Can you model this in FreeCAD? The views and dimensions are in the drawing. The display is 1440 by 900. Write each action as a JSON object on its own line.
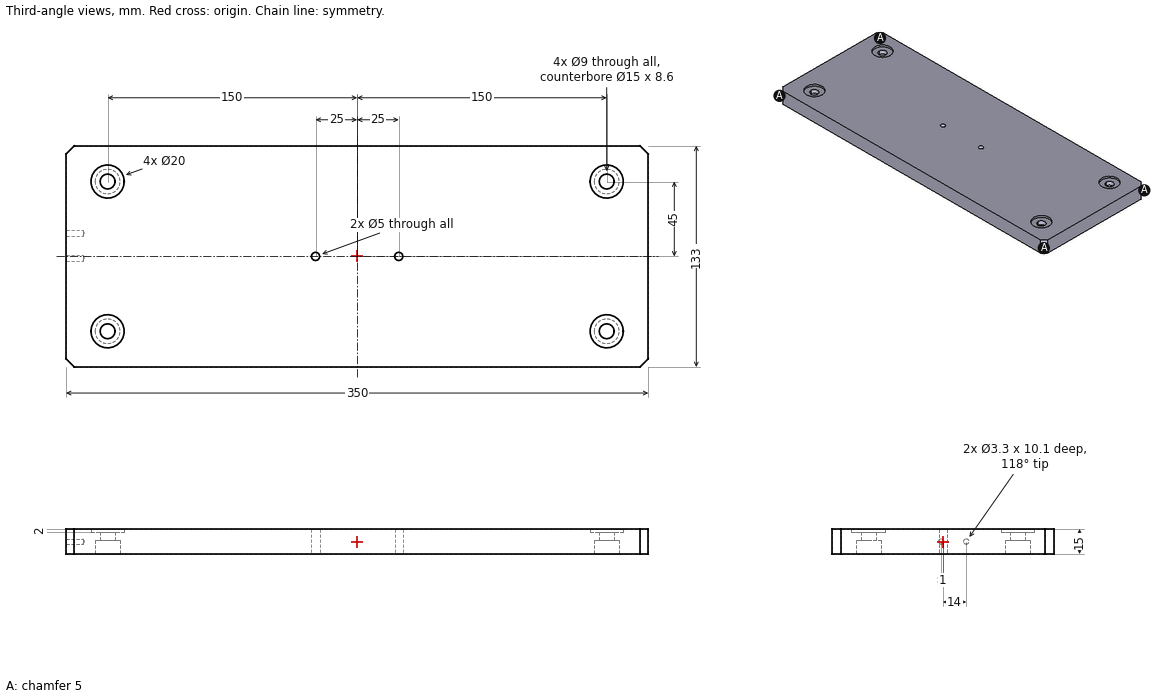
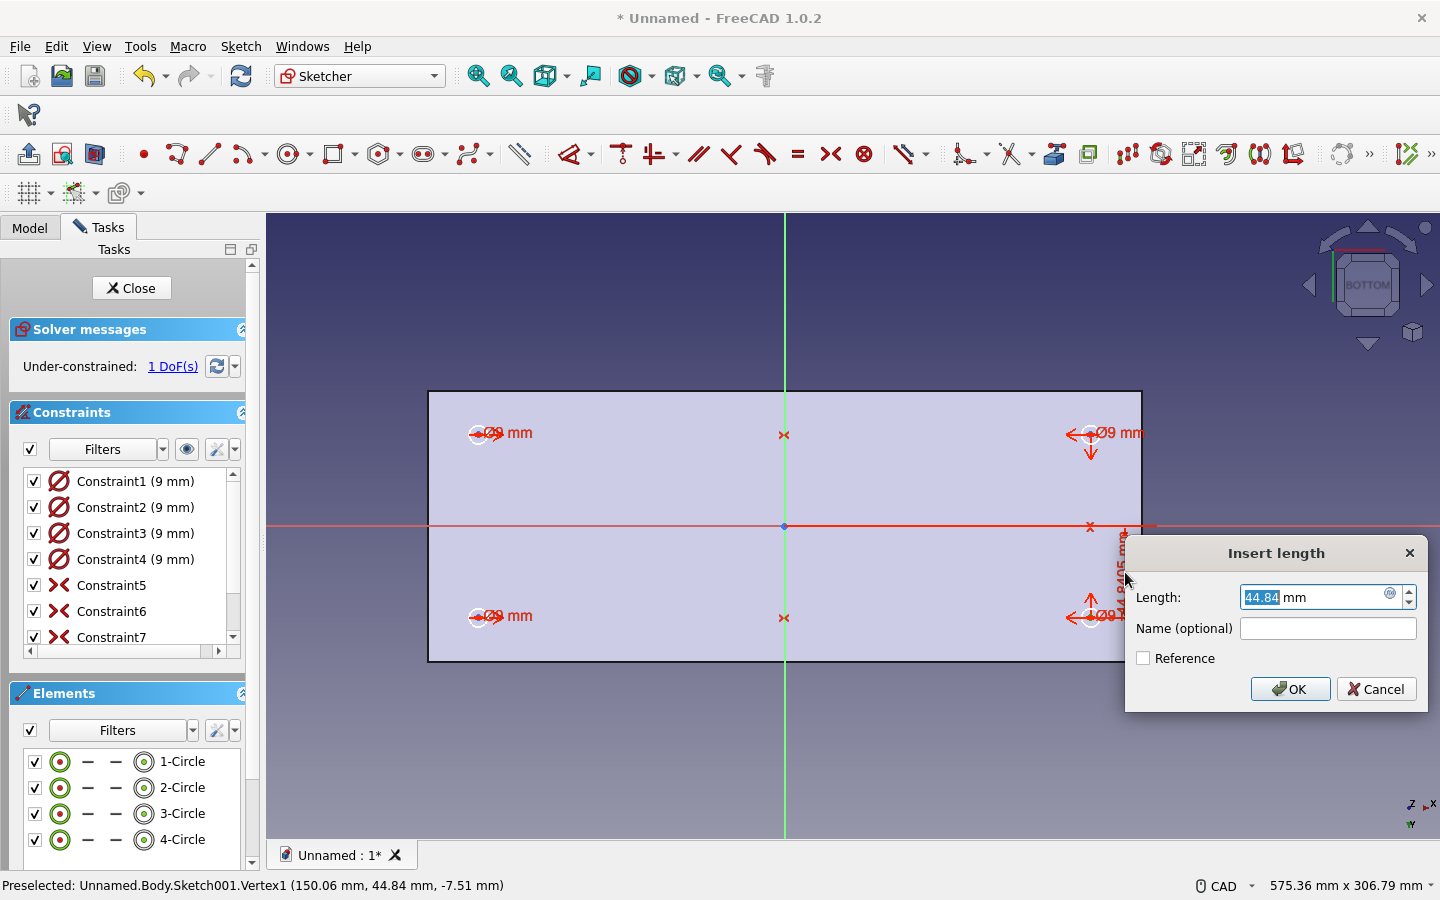
{"action": "type", "text": "45"}
{"action": "key", "text": "Return"}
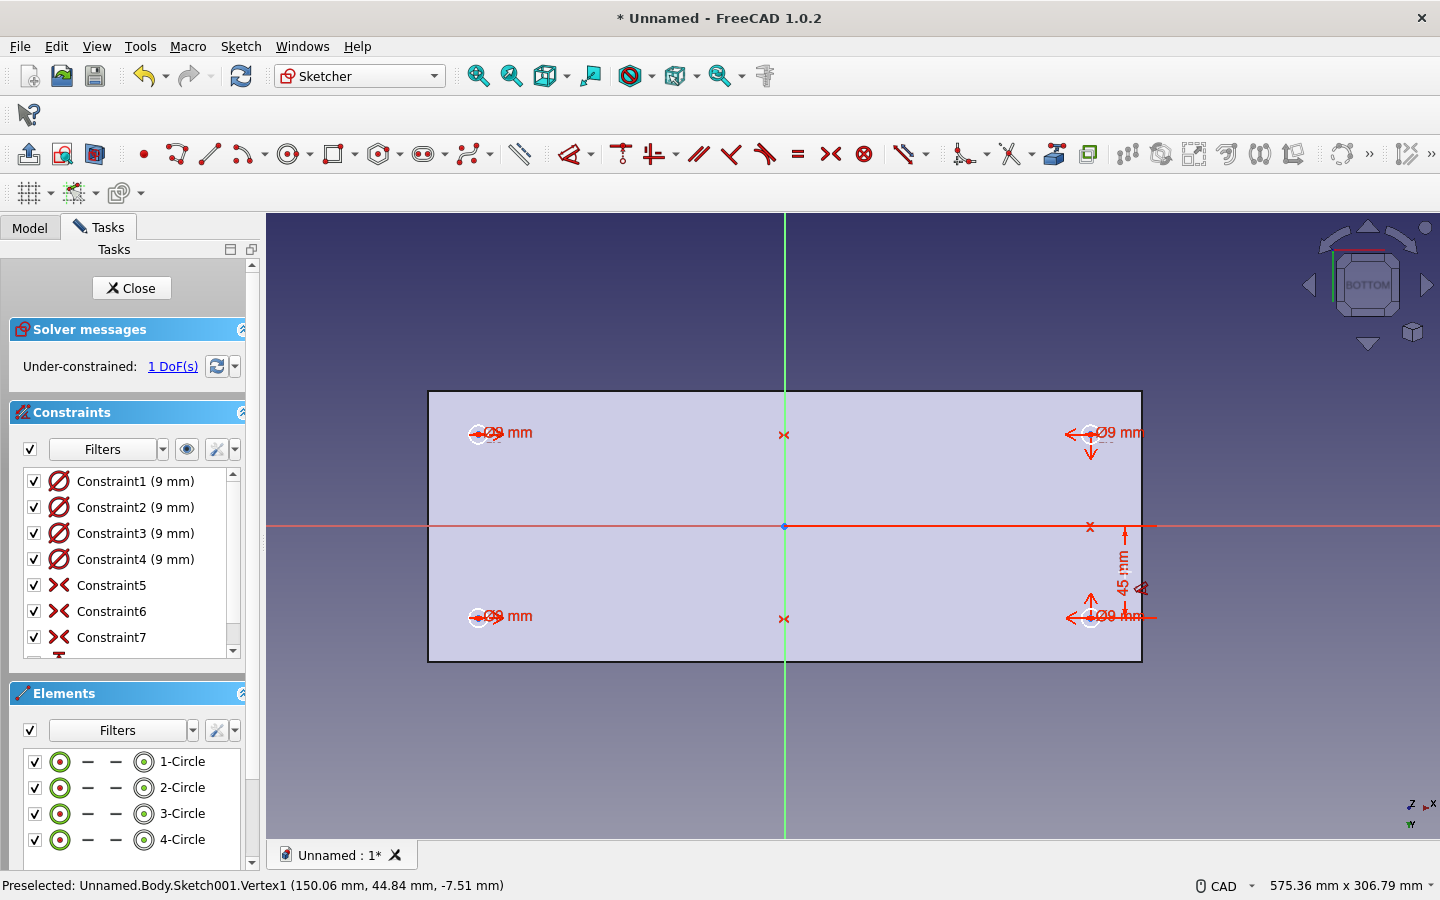
{"action": "left_click", "coordinate": [1091, 618]}
{"action": "left_click", "coordinate": [938, 652]}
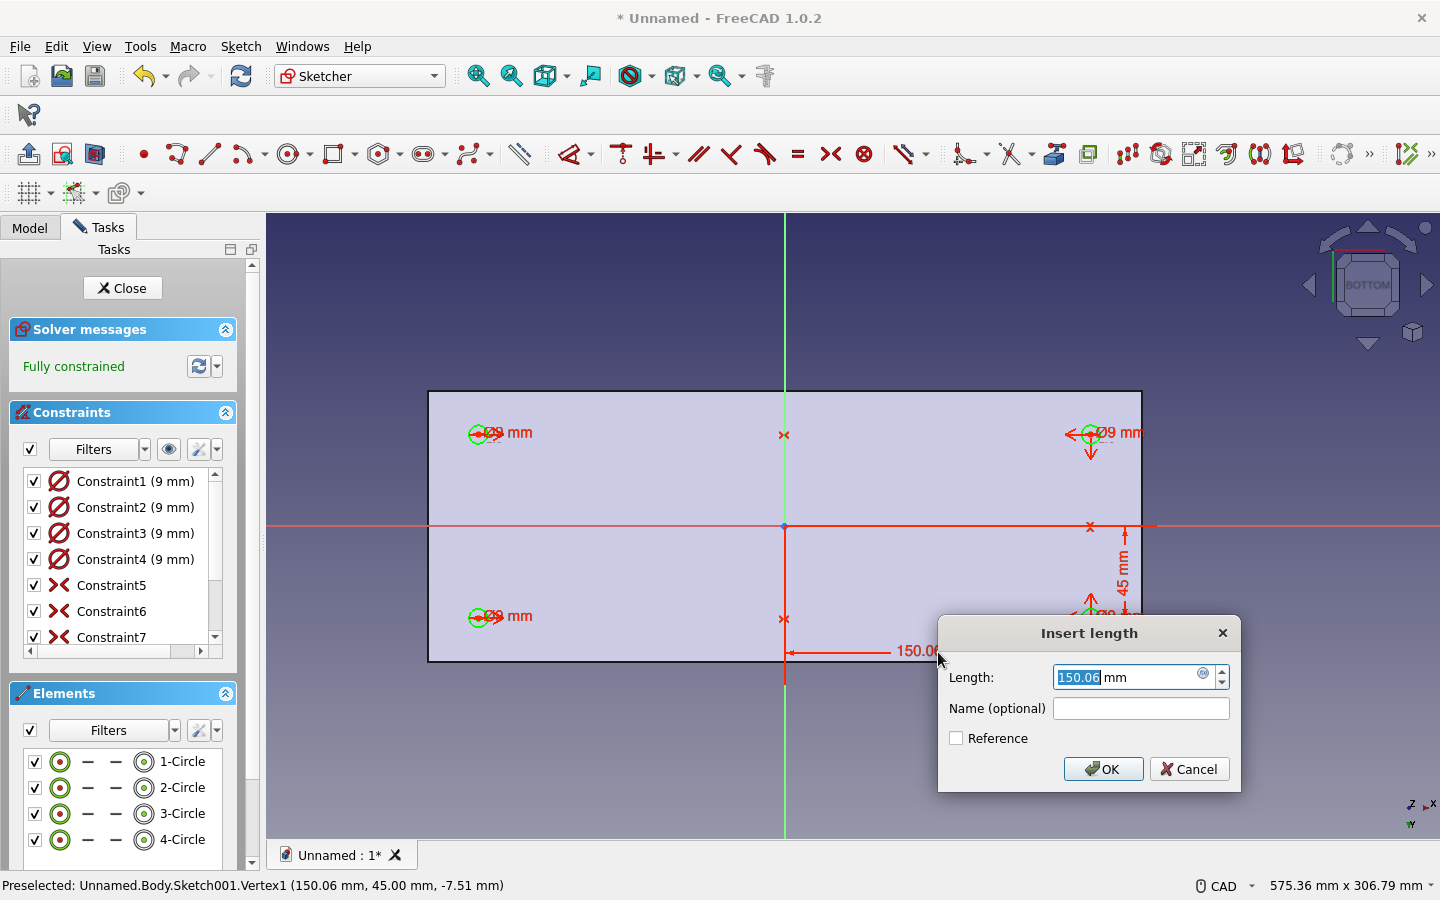
{"action": "type", "text": "150"}
{"action": "key", "text": "Return"}
{"action": "key", "text": "Escape"}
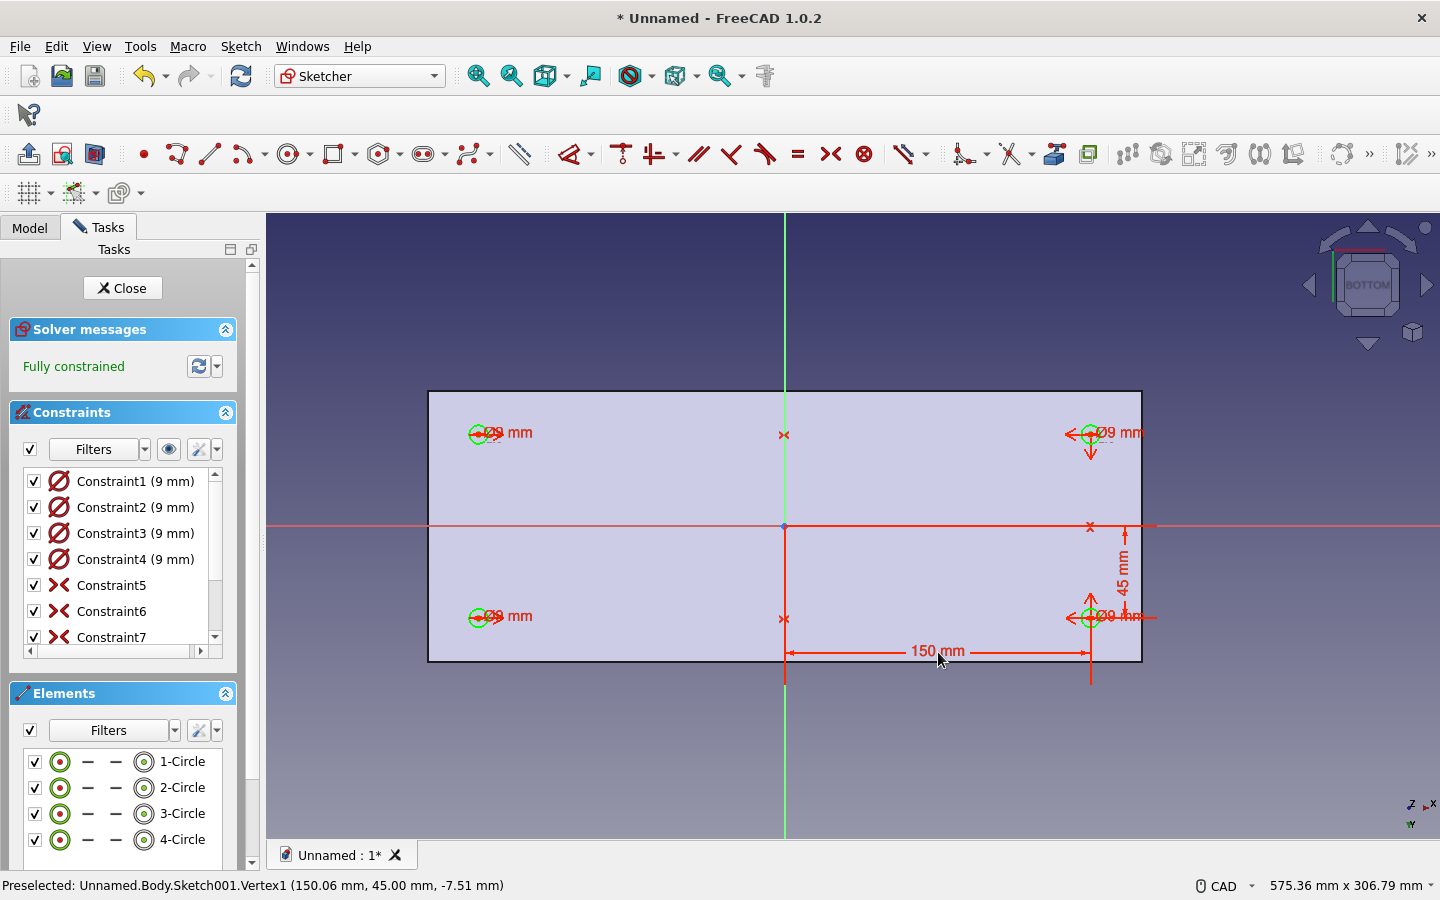
{"action": "left_click", "coordinate": [123, 288]}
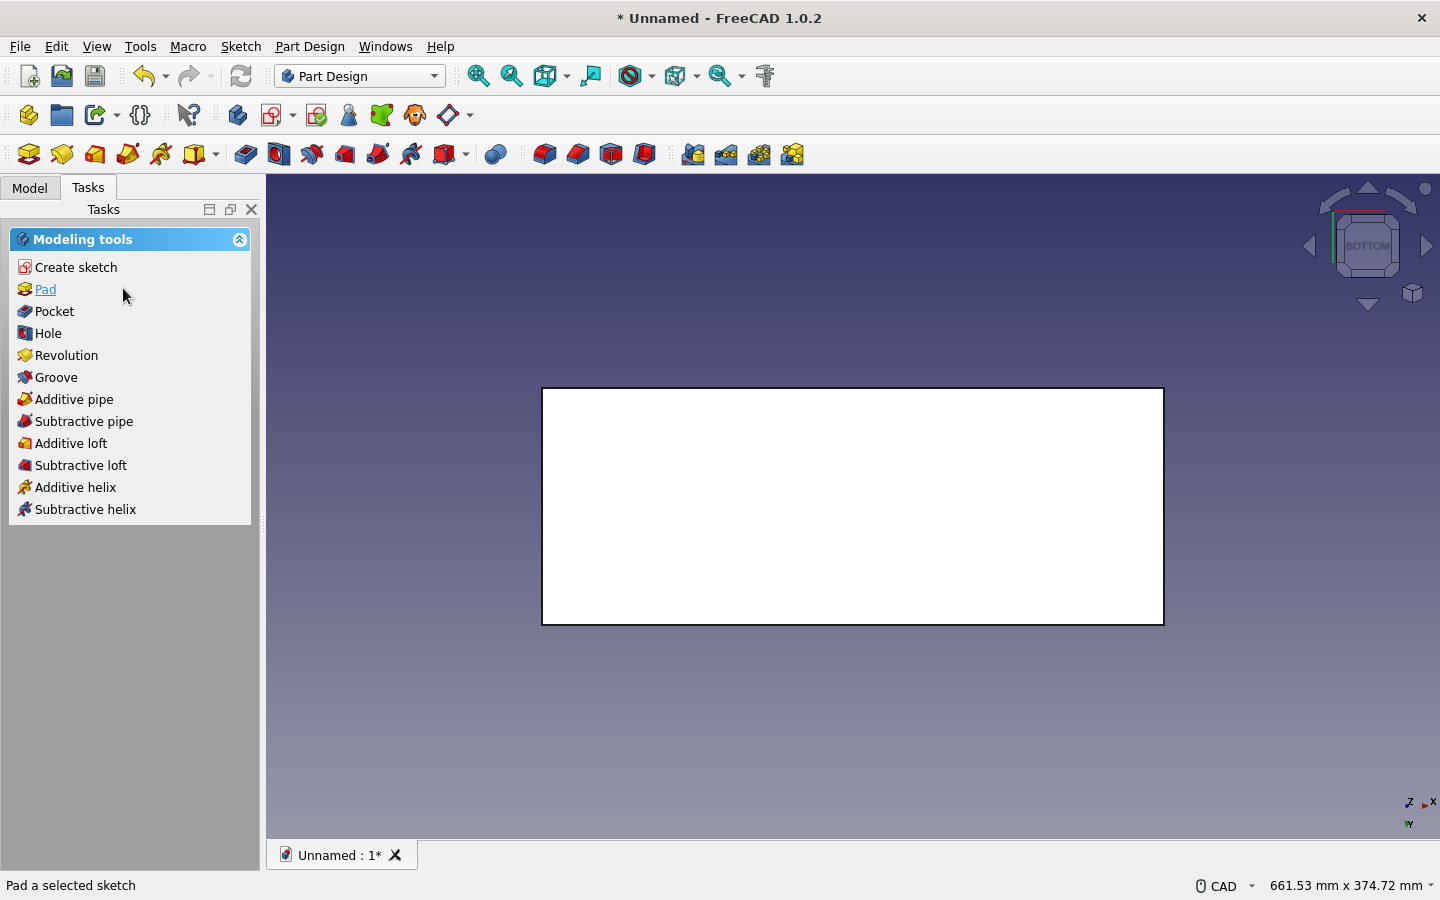
{"action": "left_click", "coordinate": [279, 154]}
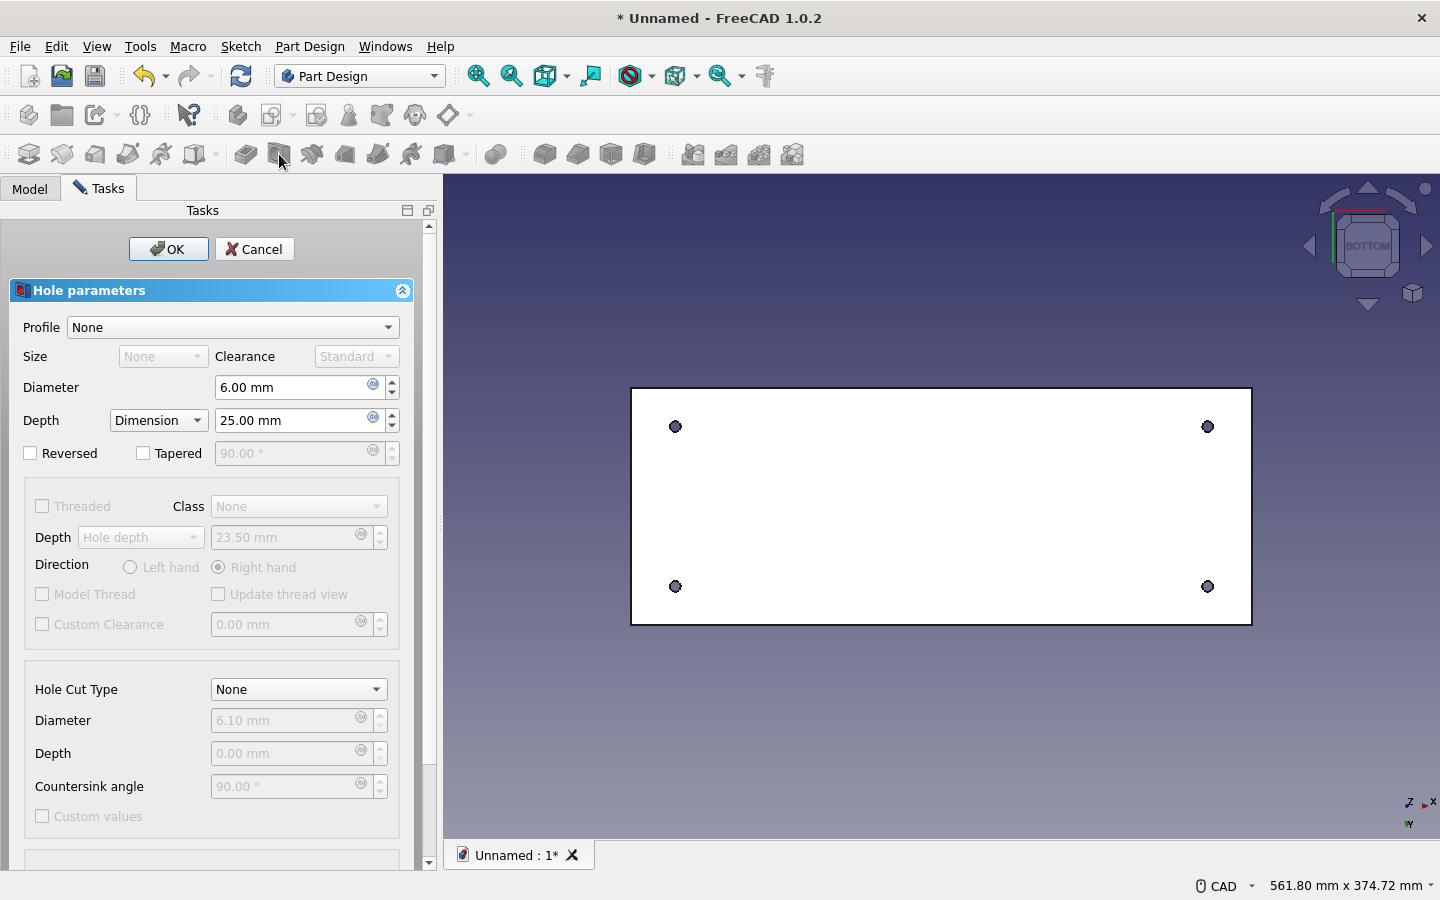
{"action": "triple_click", "coordinate": [300, 388]}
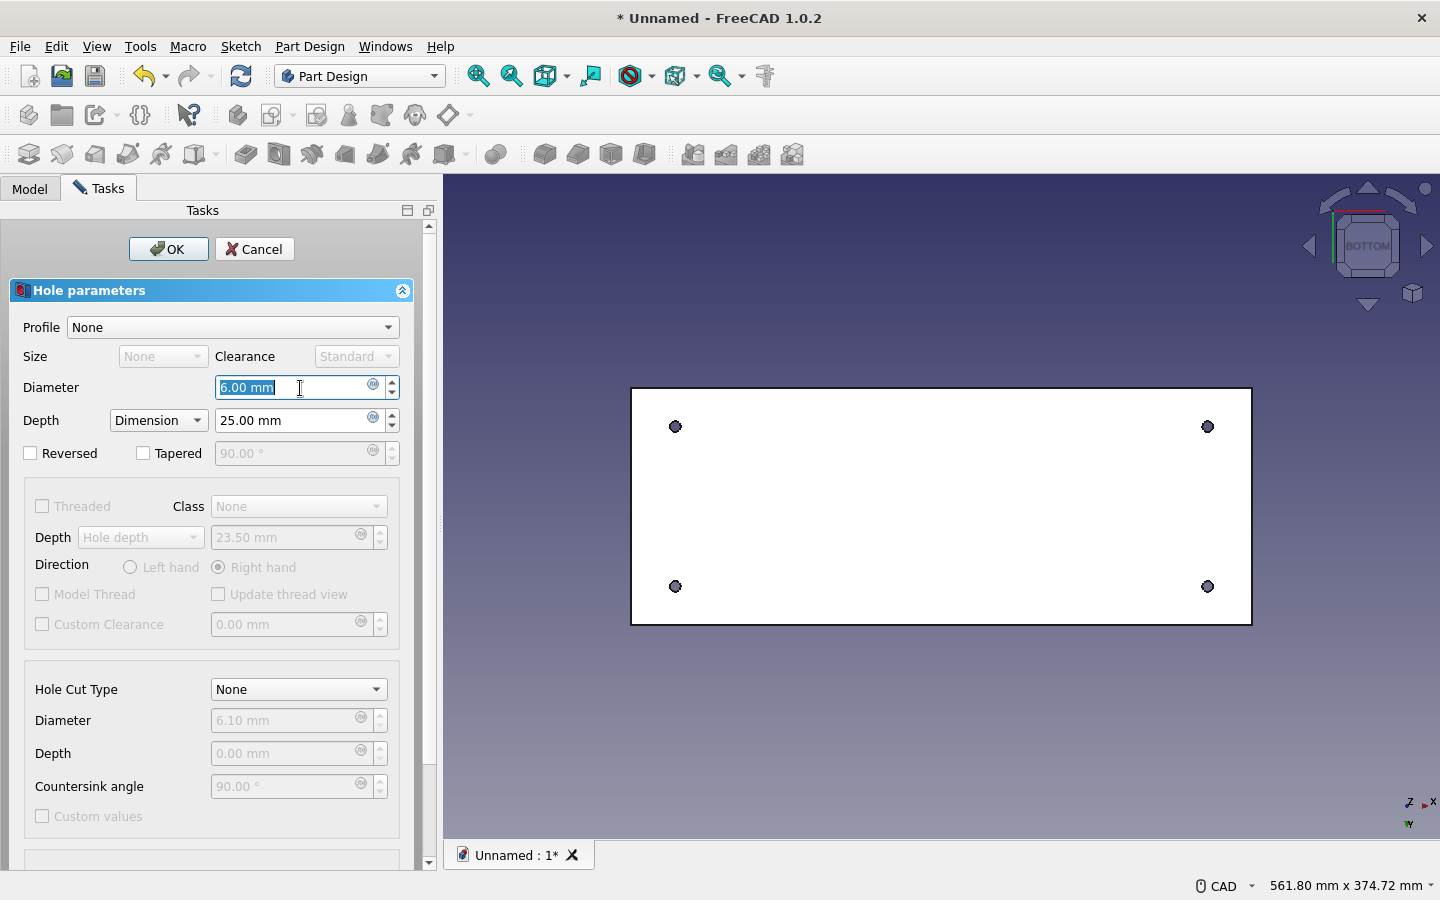
{"action": "type", "text": "9"}
{"action": "key", "text": "Tab"}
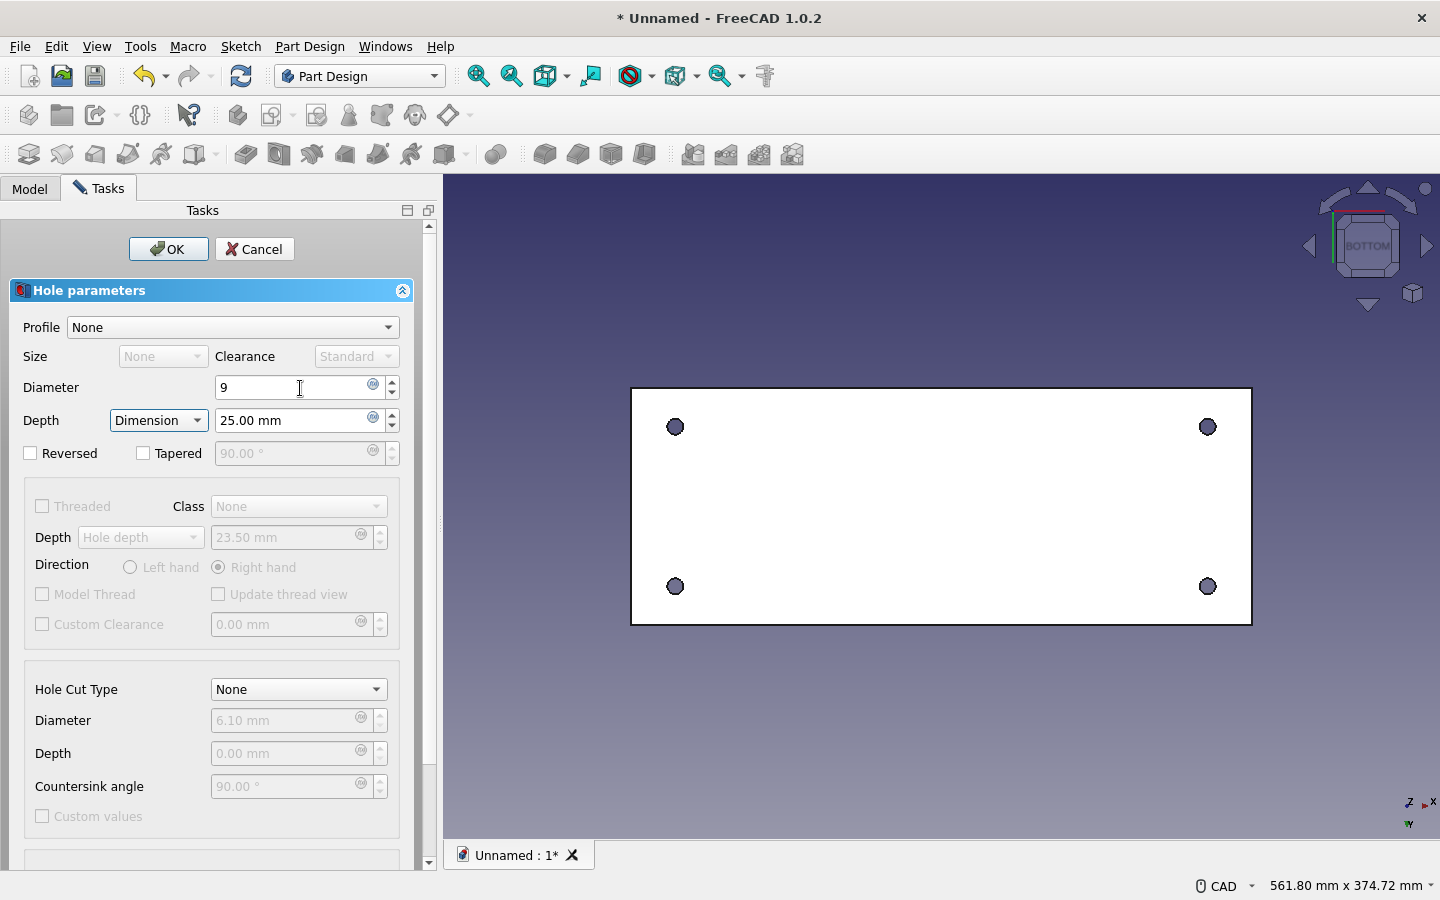
{"action": "left_click", "coordinate": [160, 420]}